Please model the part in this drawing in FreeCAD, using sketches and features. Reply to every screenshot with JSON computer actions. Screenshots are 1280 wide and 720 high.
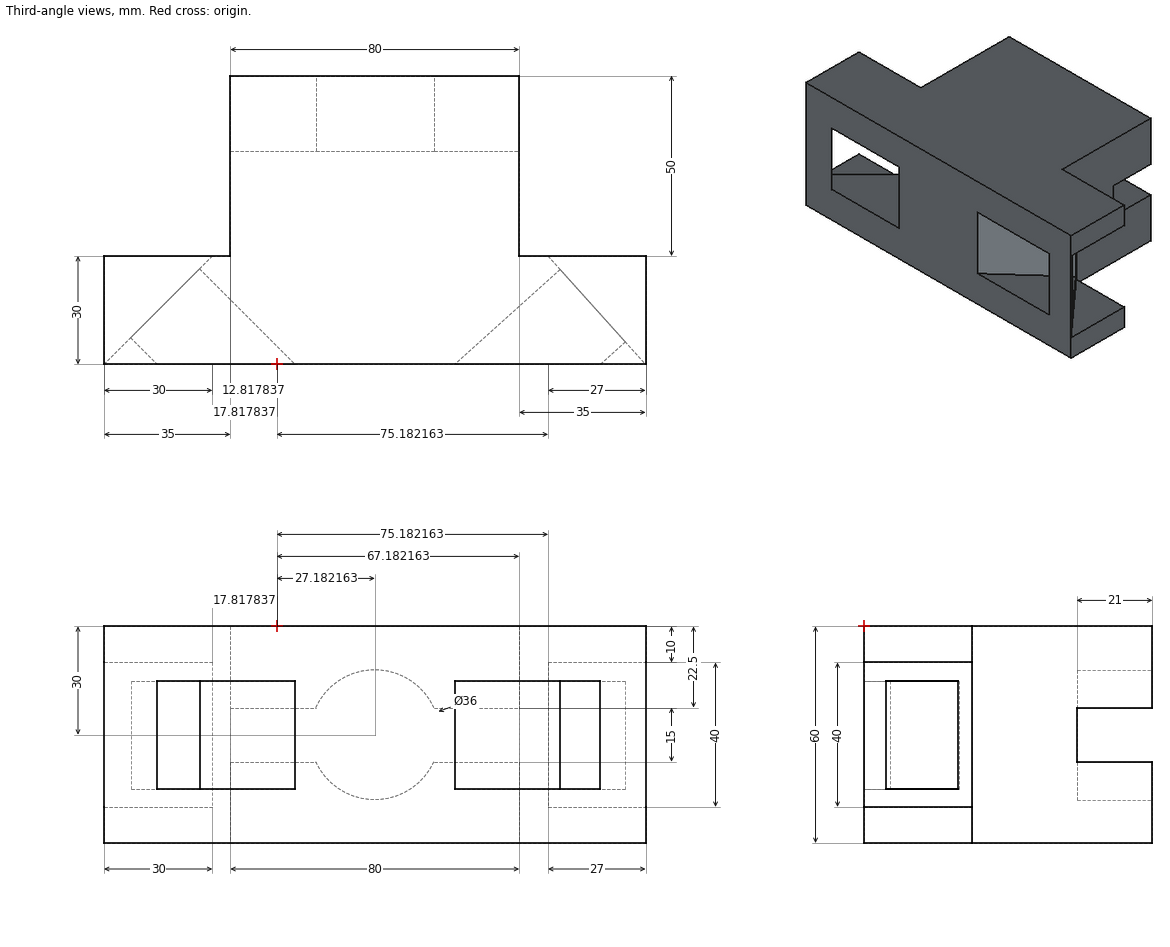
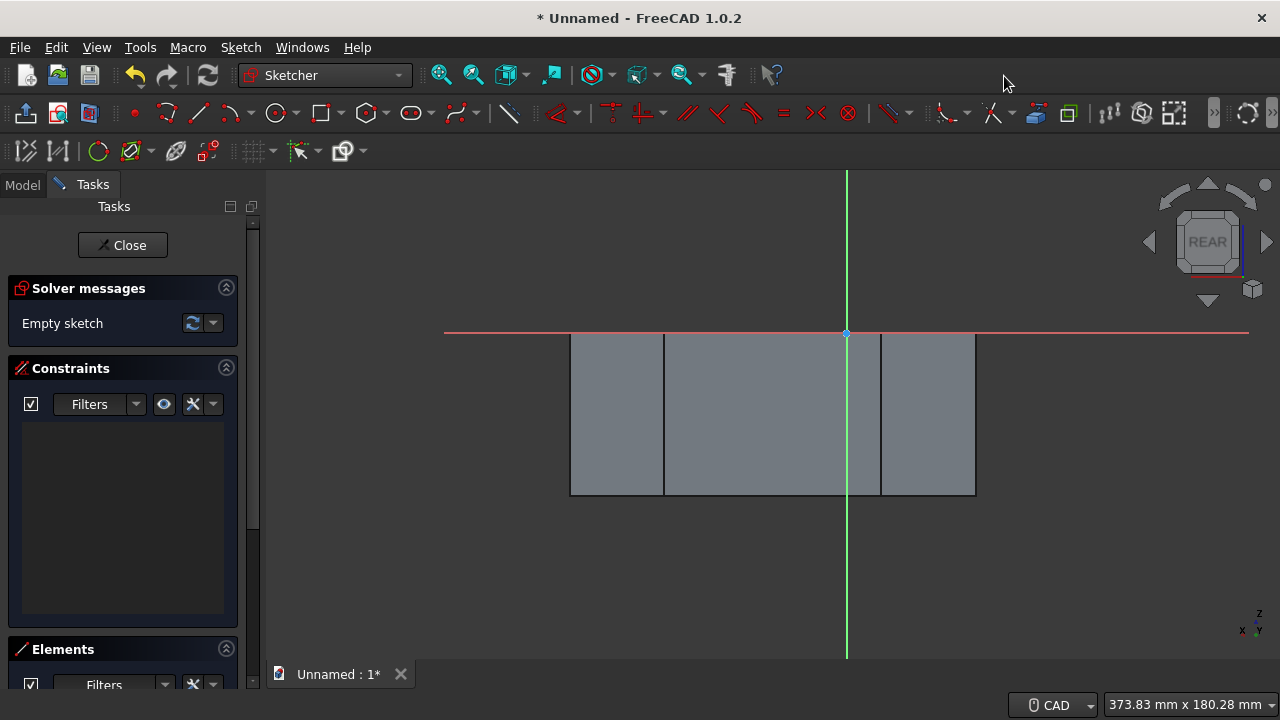
{"action": "scroll", "coordinate": [852, 385], "scroll_direction": "up", "scroll_amount": 4}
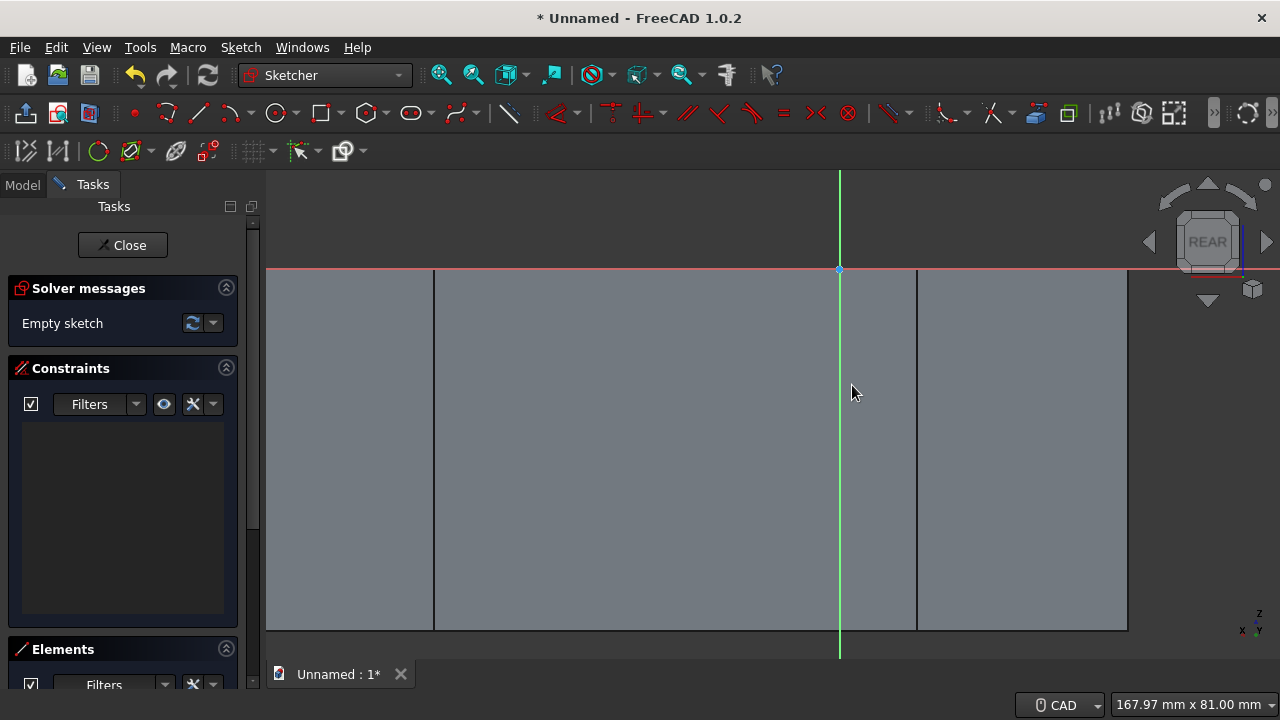
{"action": "left_click", "coordinate": [276, 114]}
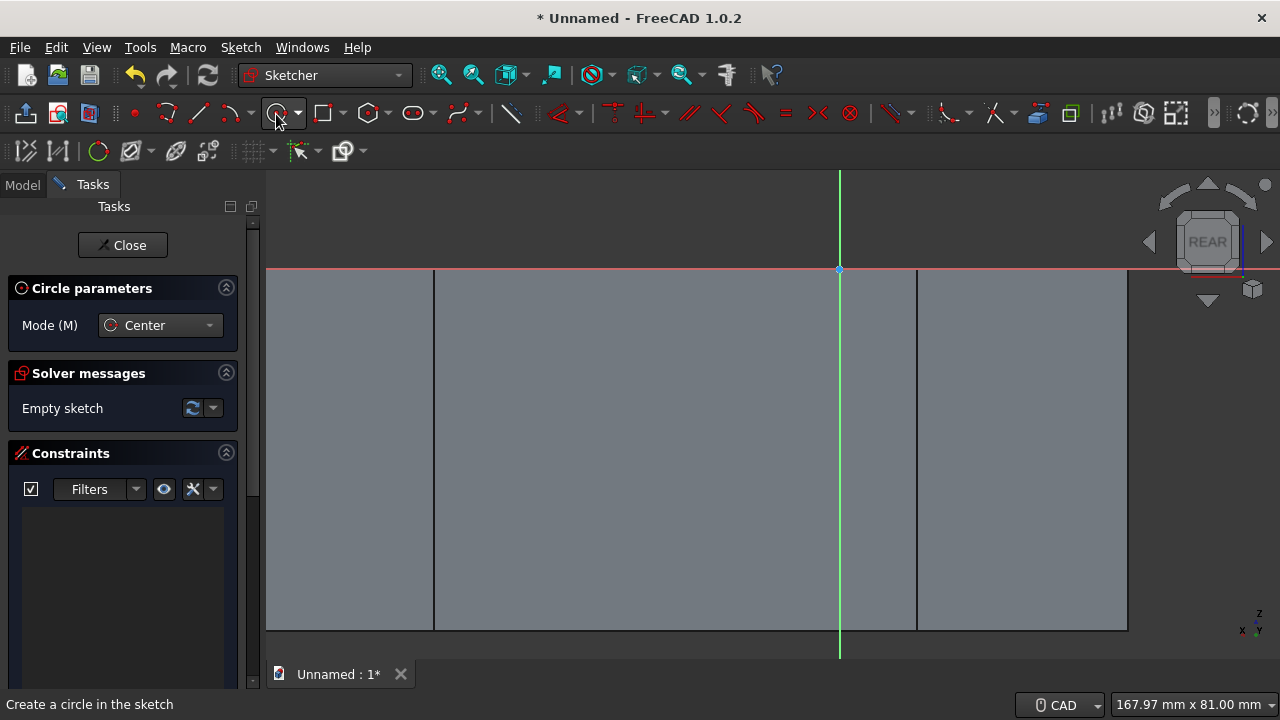
{"action": "left_click", "coordinate": [675, 450]}
{"action": "left_click", "coordinate": [752, 373]}
{"action": "key", "text": "Escape"}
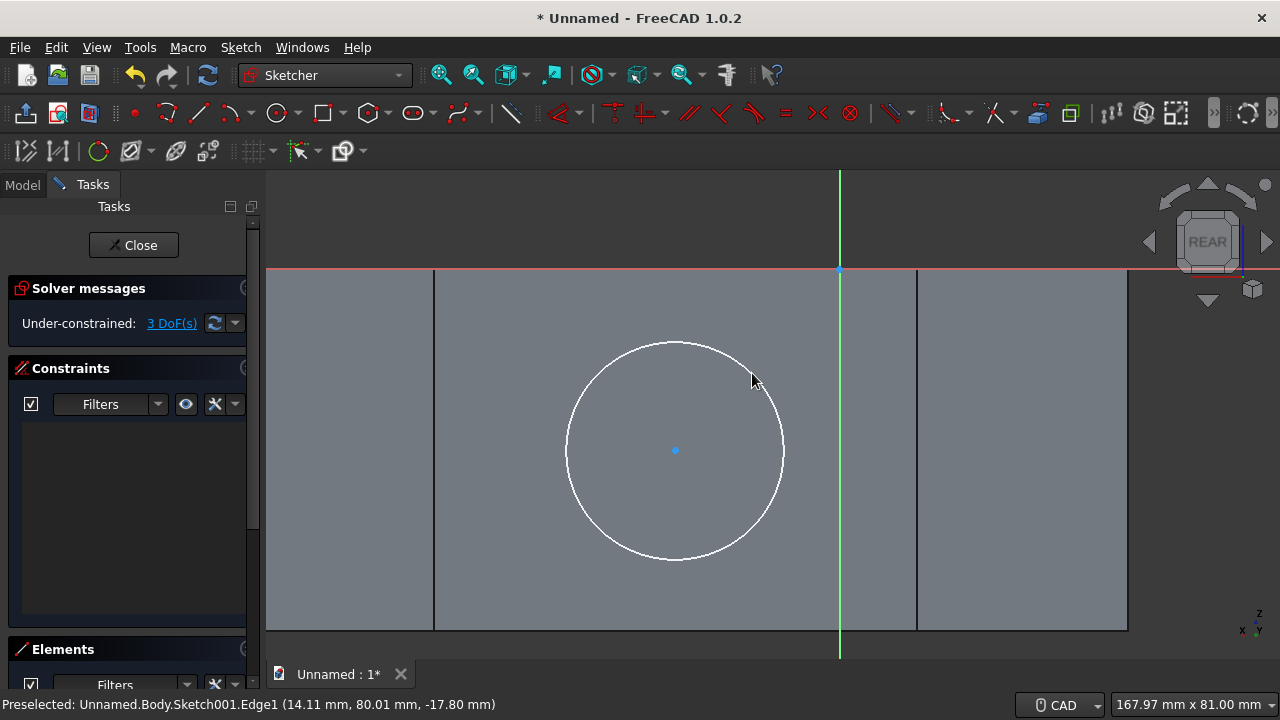
{"action": "left_click", "coordinate": [558, 114]}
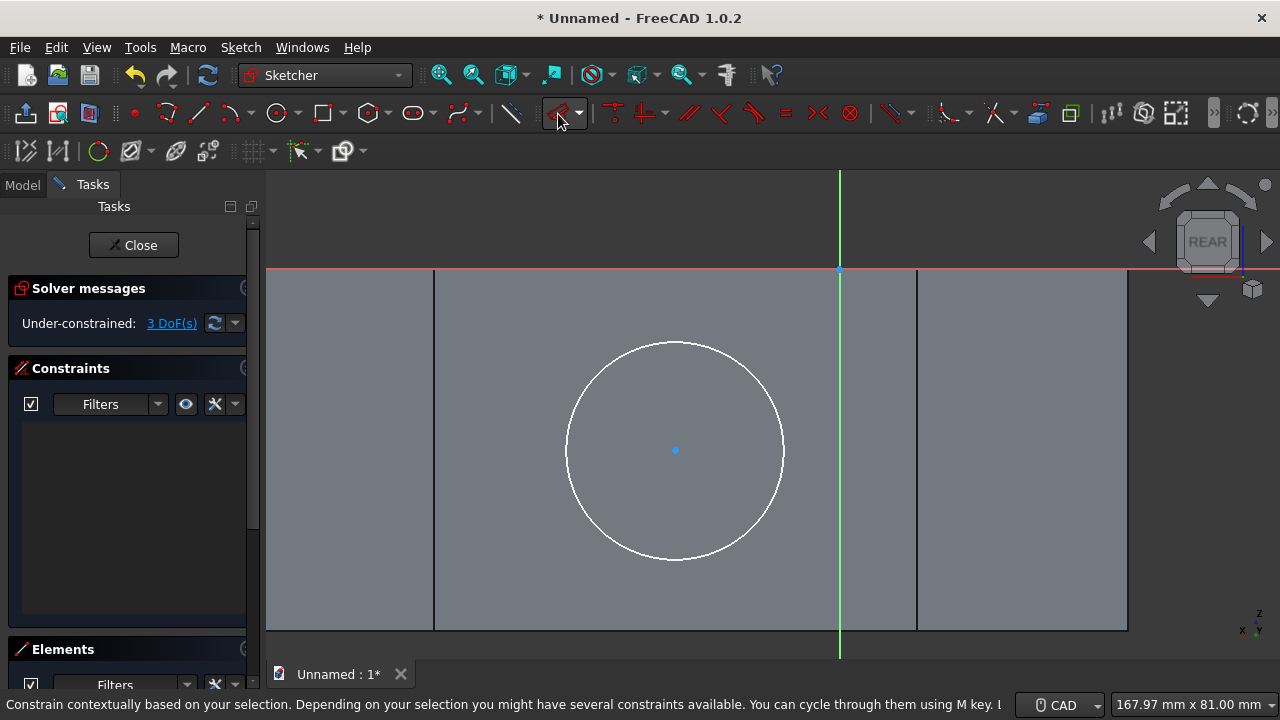
{"action": "left_click", "coordinate": [752, 374]}
{"action": "left_click", "coordinate": [775, 351]}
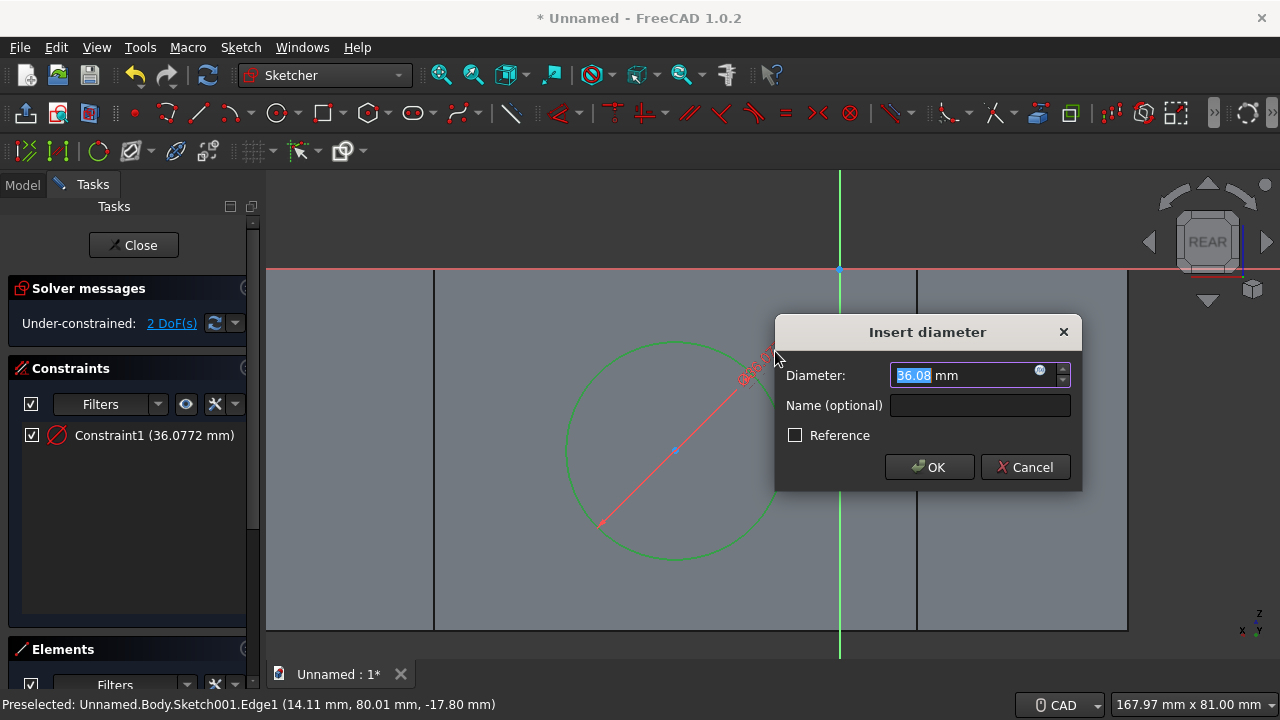
{"action": "type", "text": "36"}
{"action": "key", "text": "Return"}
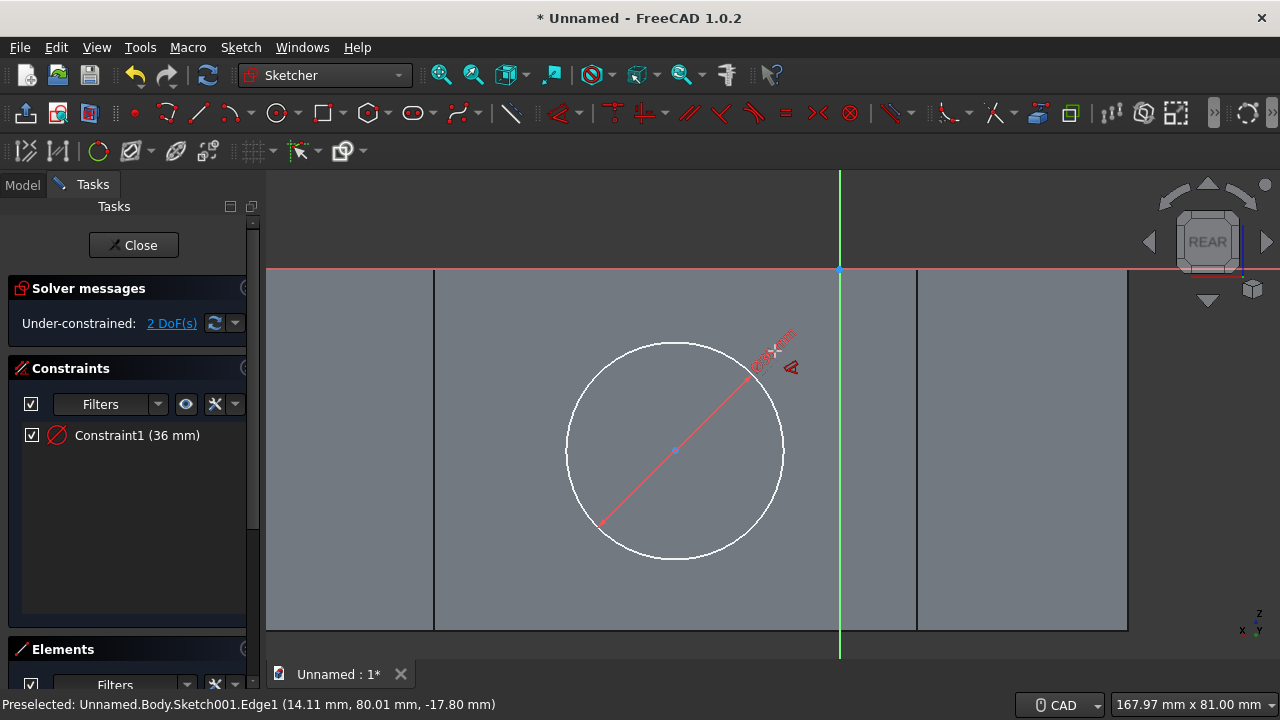
{"action": "left_click", "coordinate": [675, 451]}
{"action": "left_click", "coordinate": [874, 360]}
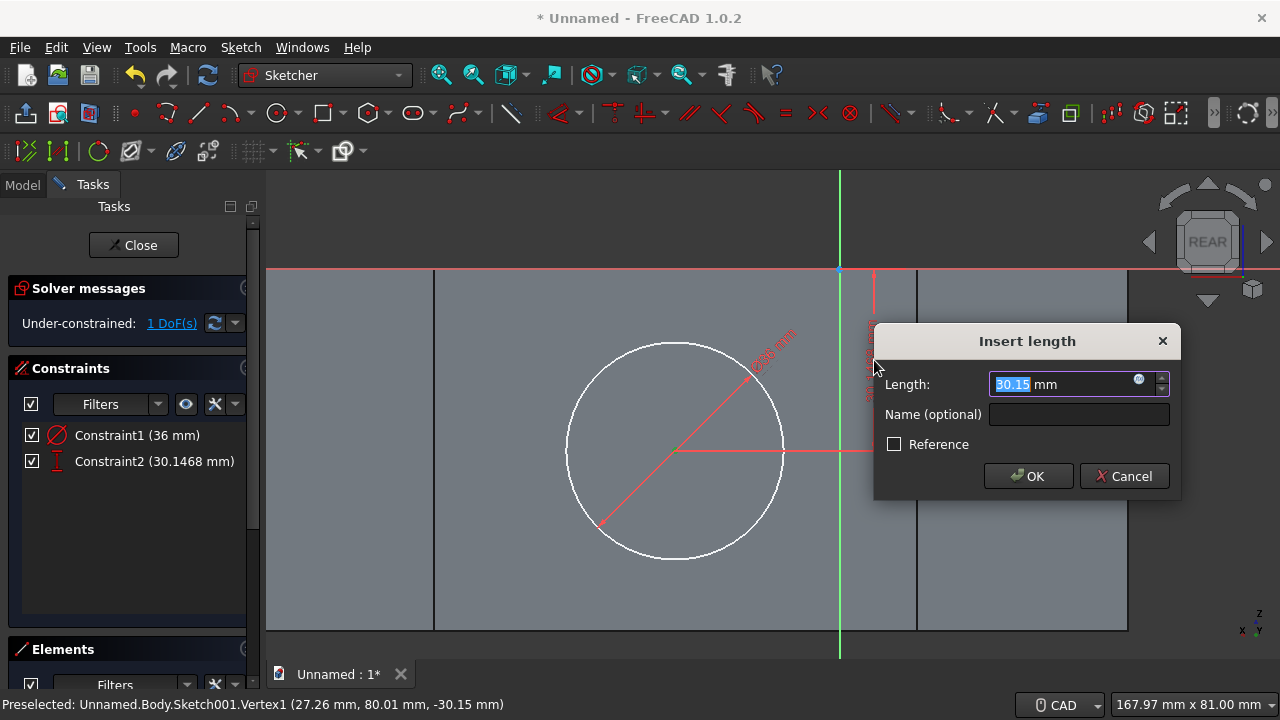
{"action": "type", "text": "30"}
{"action": "key", "text": "Return"}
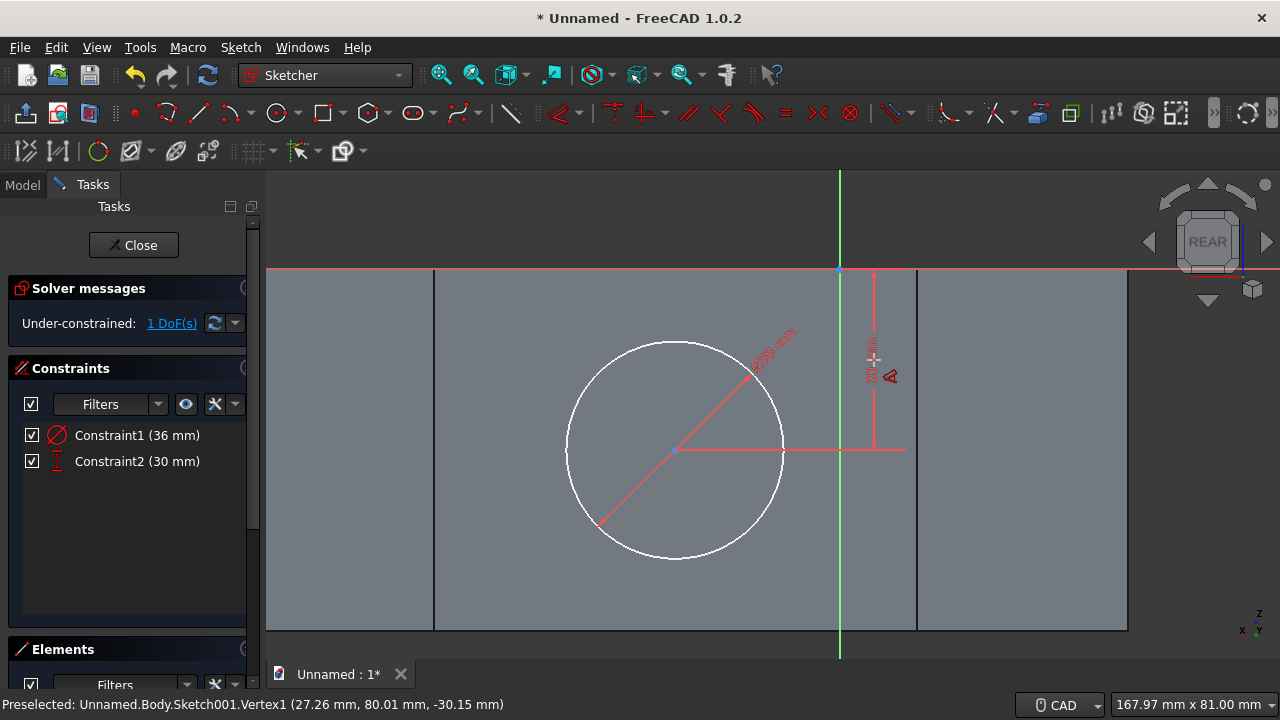
{"action": "left_click", "coordinate": [675, 450]}
{"action": "left_click", "coordinate": [757, 235]}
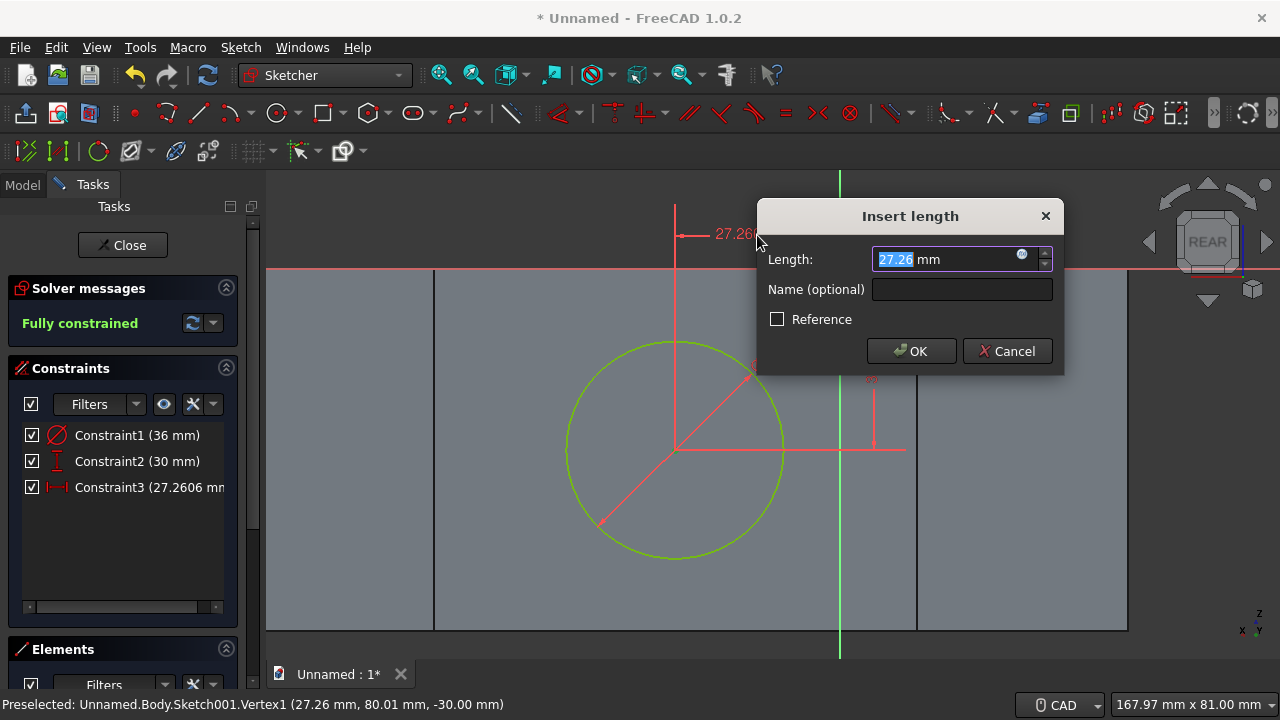
{"action": "type", "text": "27.182163"}
{"action": "key", "text": "Return"}
{"action": "key", "text": "Escape"}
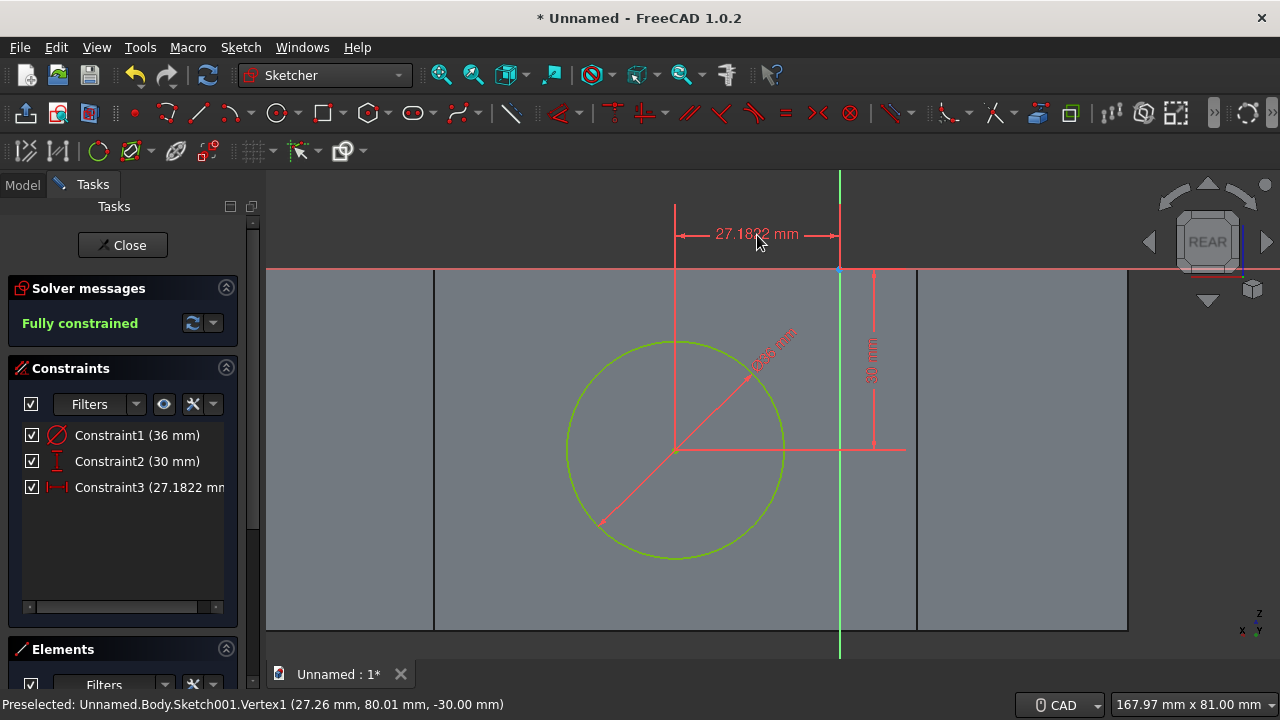
{"action": "left_click", "coordinate": [123, 245]}